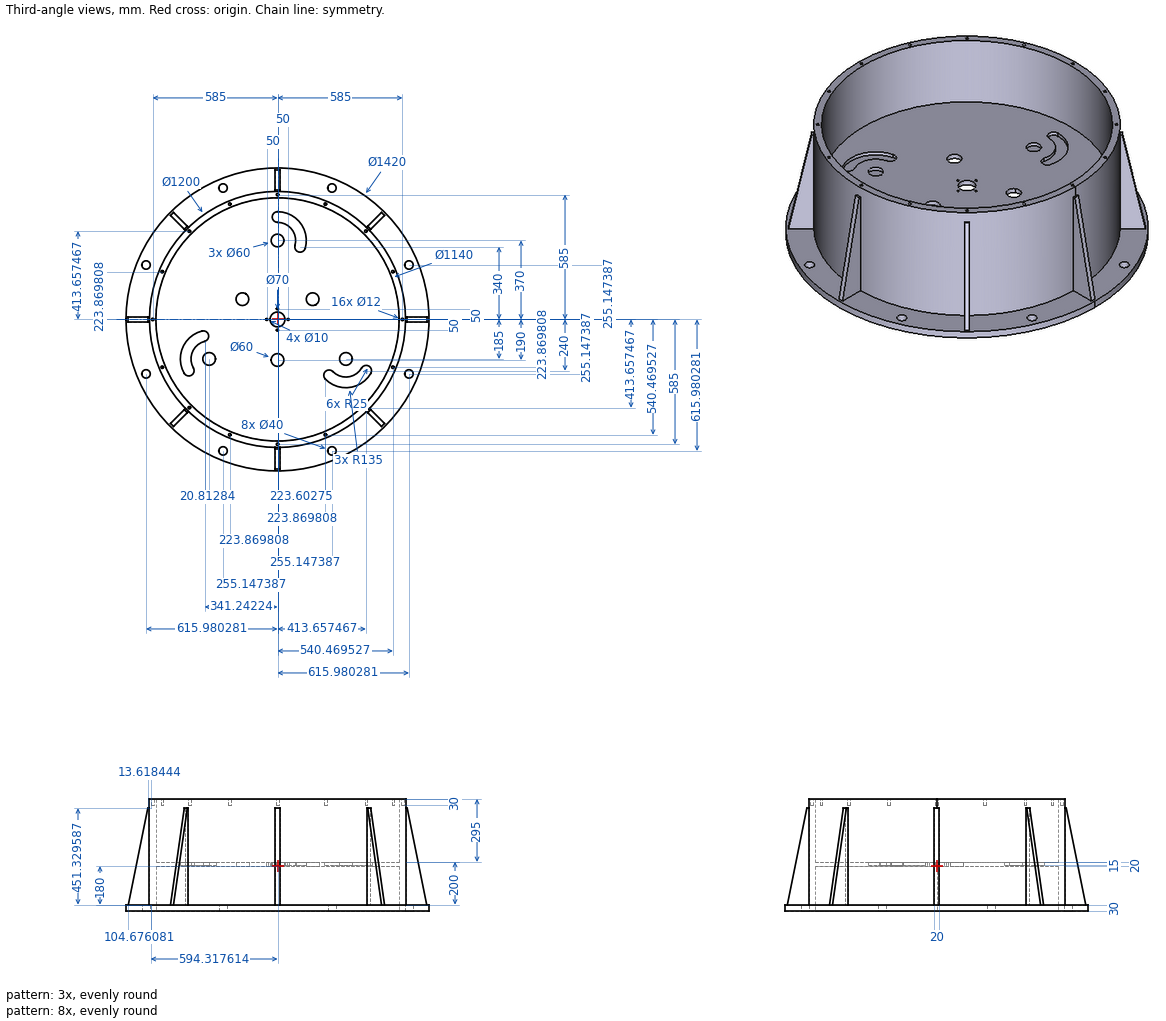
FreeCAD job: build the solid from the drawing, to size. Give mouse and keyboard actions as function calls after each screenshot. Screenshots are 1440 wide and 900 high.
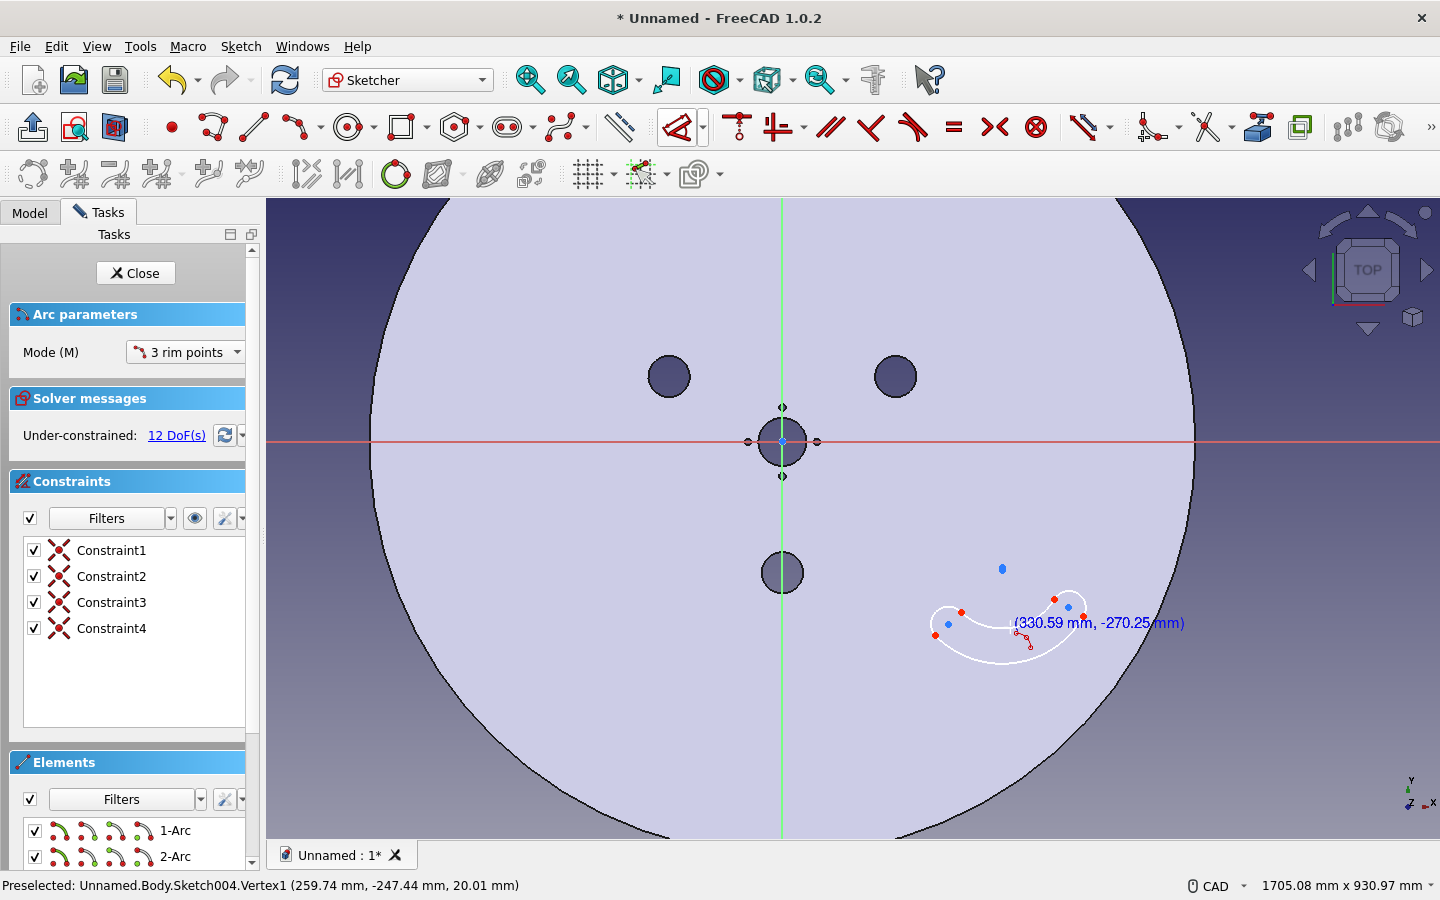
click(547, 513)
click(539, 479)
click(560, 492)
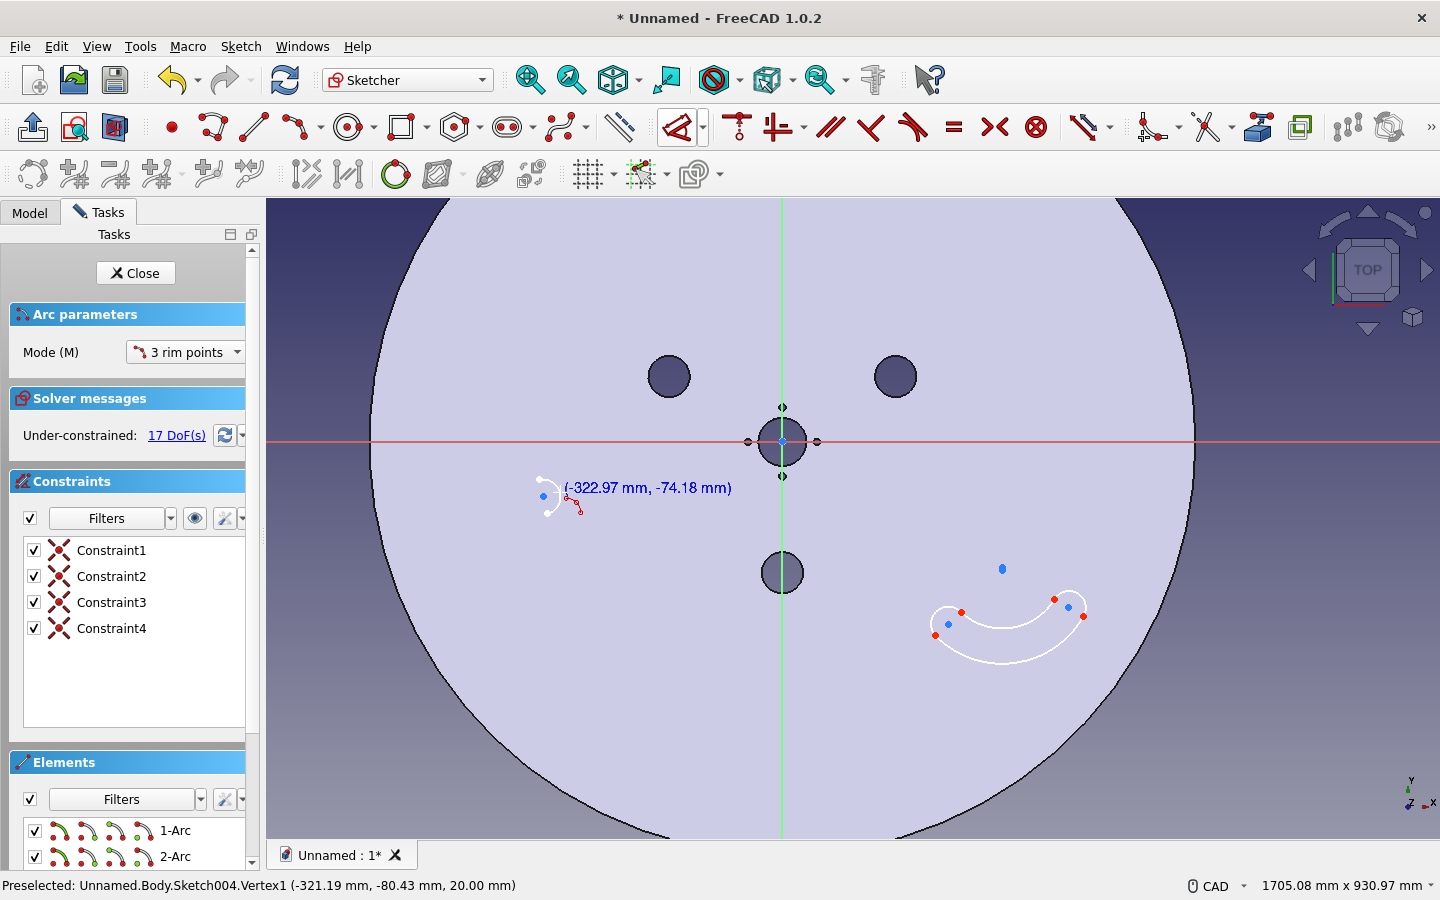
click(539, 480)
click(481, 616)
click(476, 533)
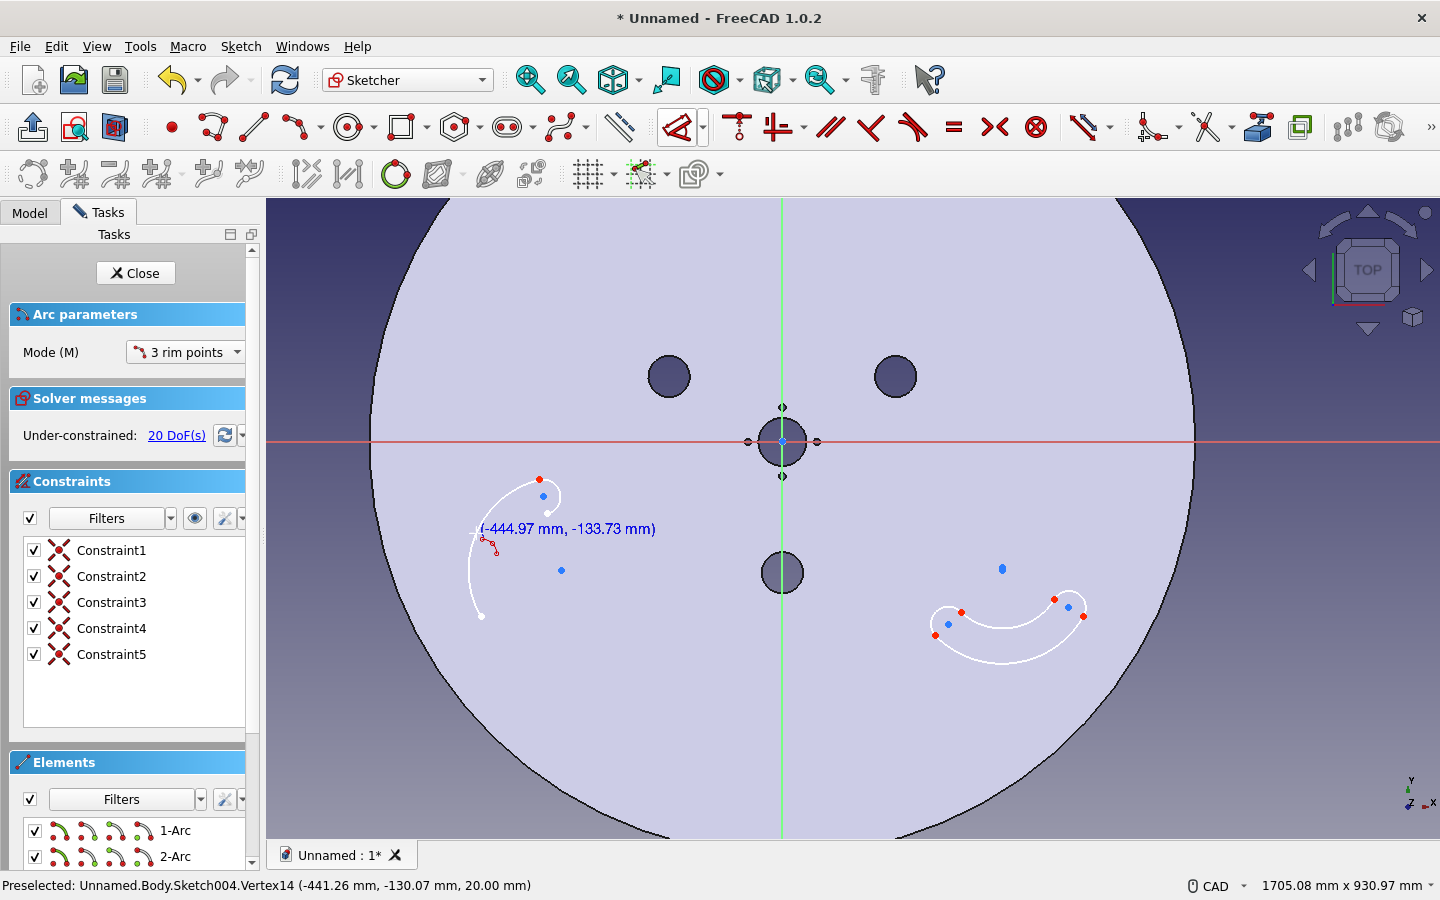
click(481, 617)
click(511, 599)
click(505, 622)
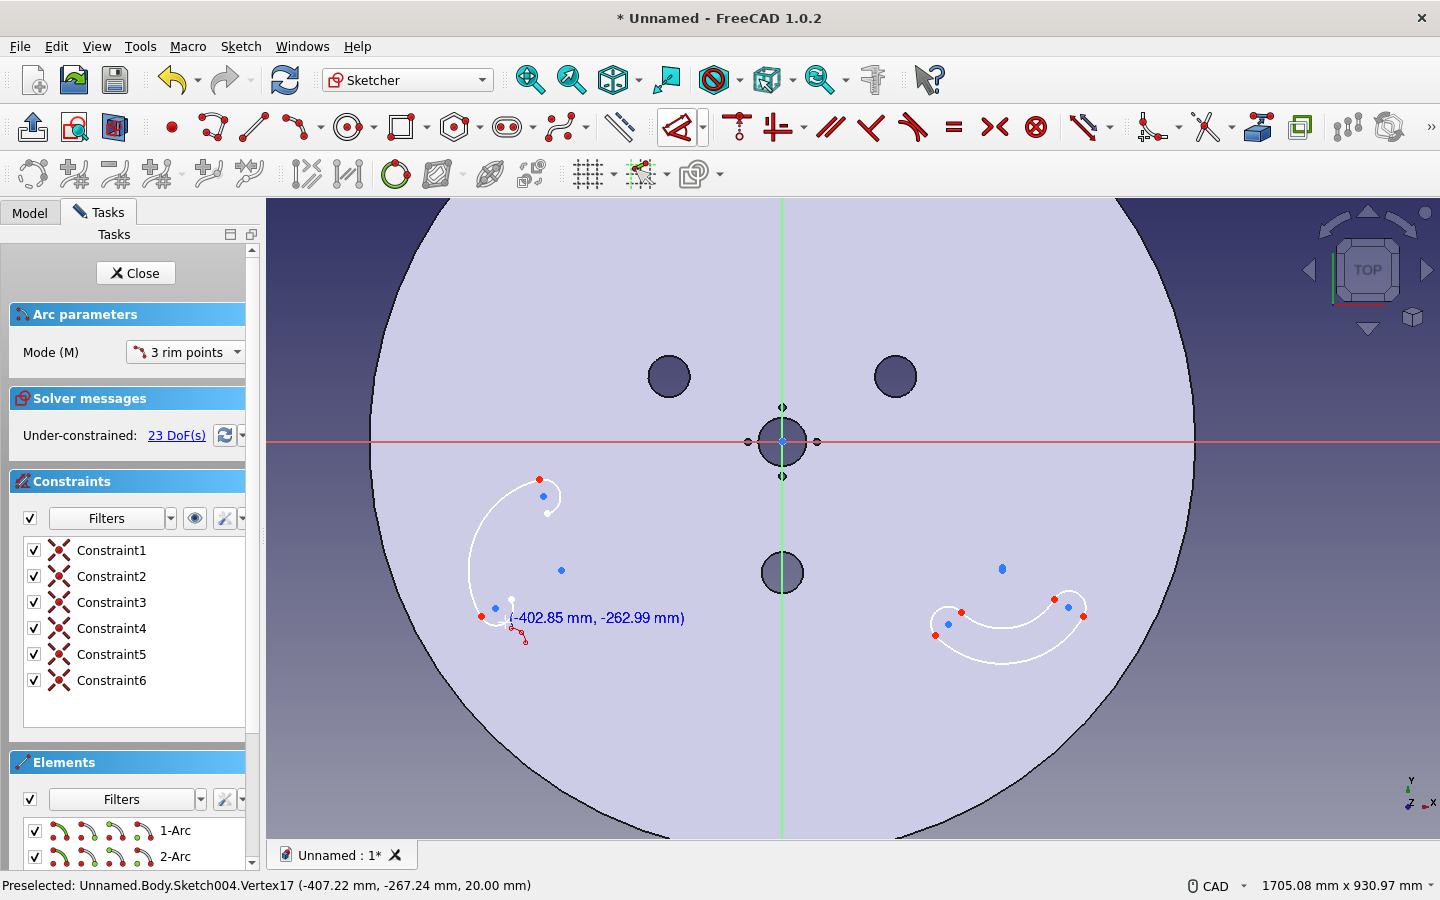
click(511, 600)
click(547, 514)
click(508, 547)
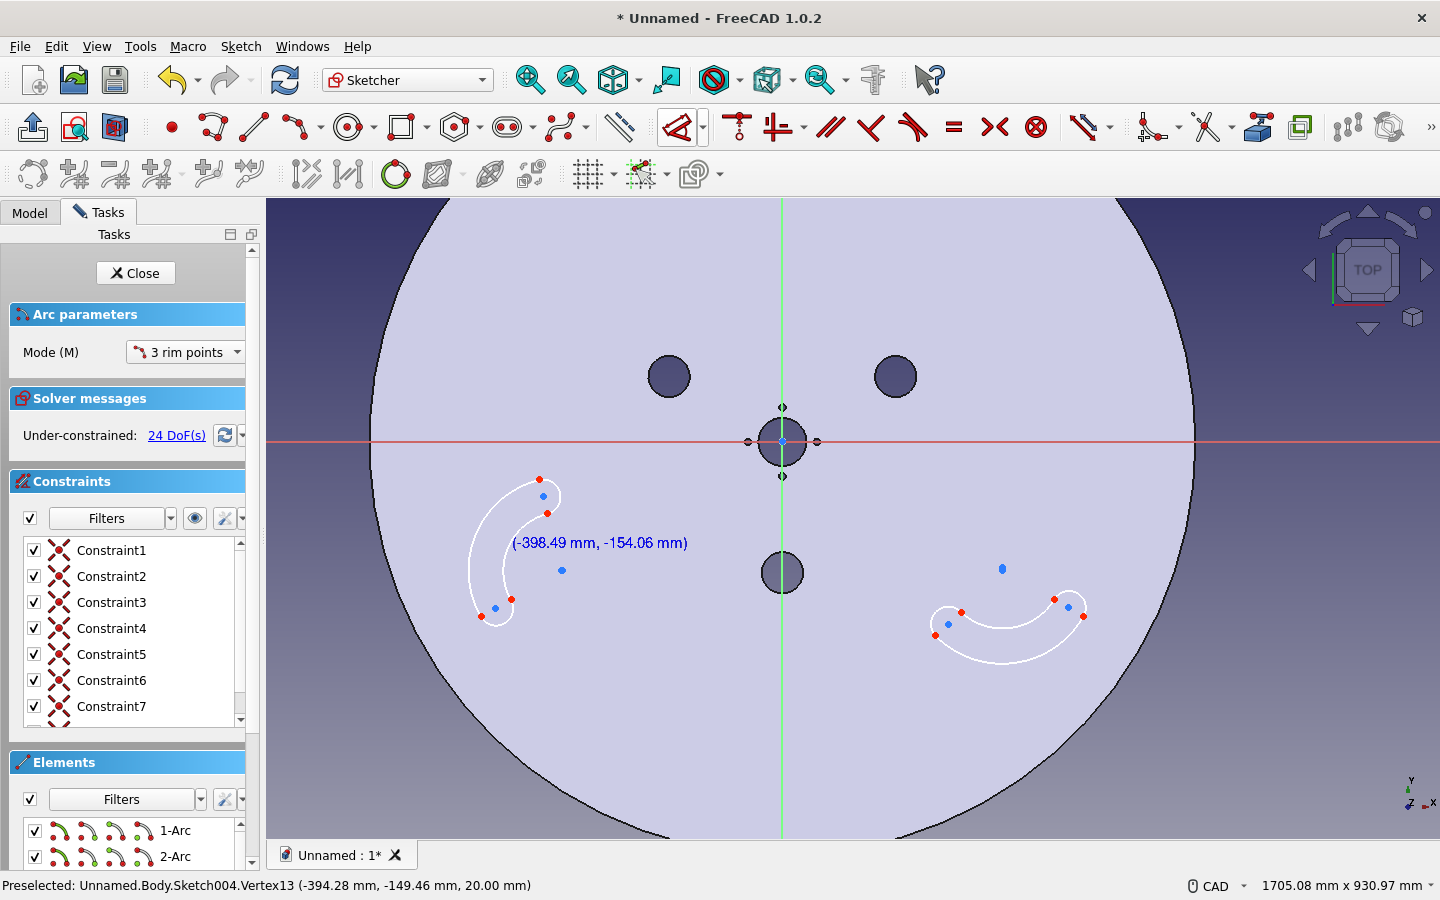
scroll(794, 804, down, 2)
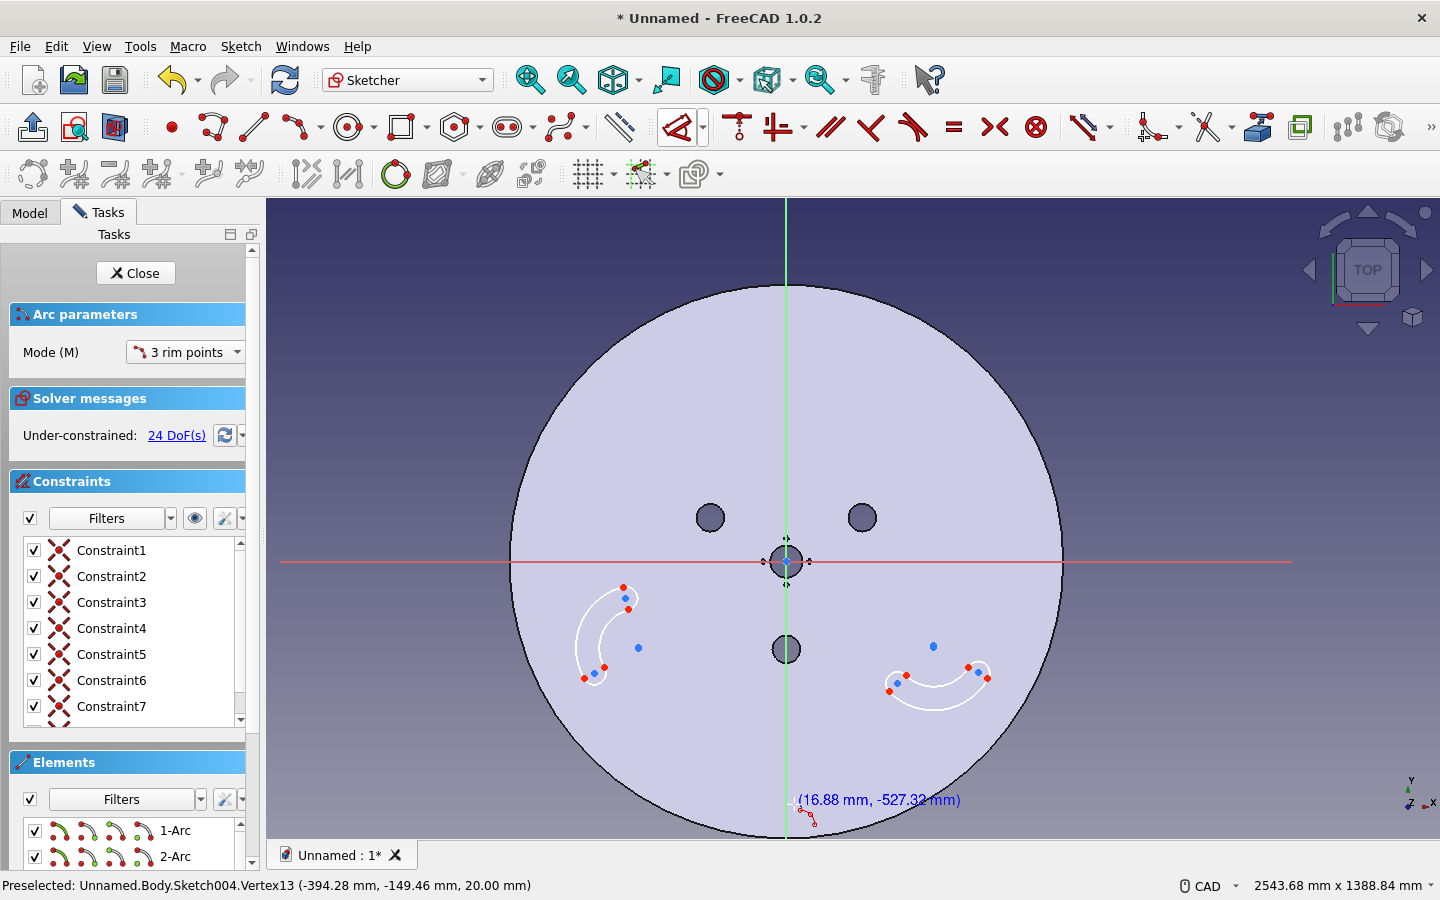
click(824, 402)
click(846, 408)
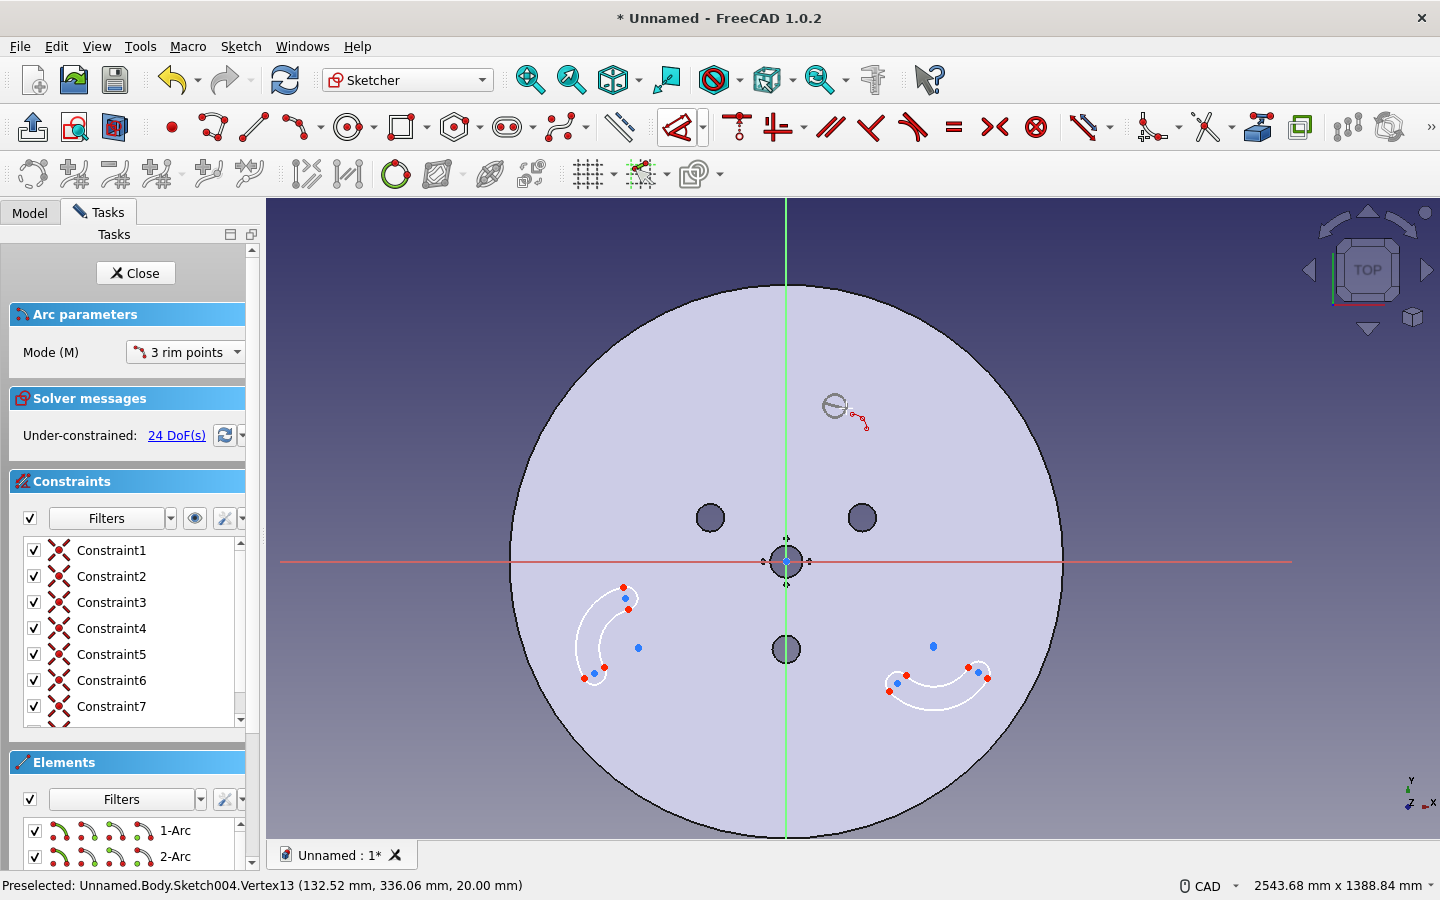
scroll(832, 416, up, 2)